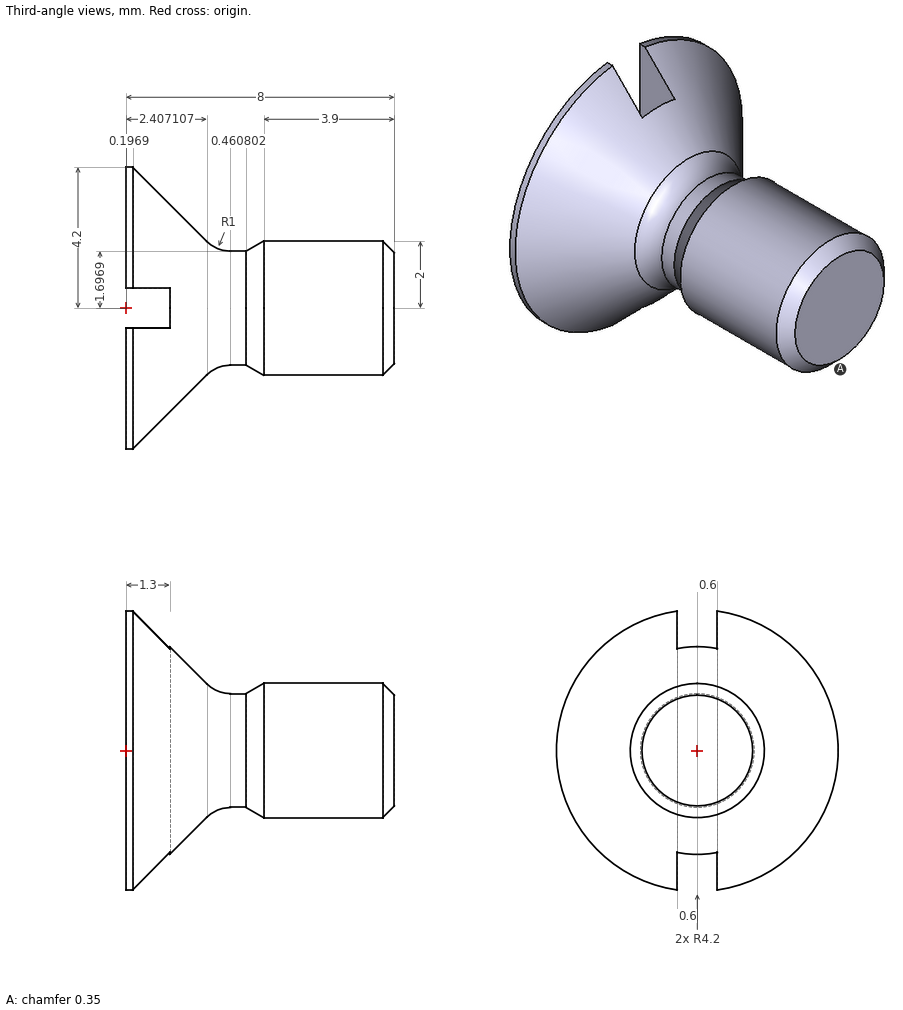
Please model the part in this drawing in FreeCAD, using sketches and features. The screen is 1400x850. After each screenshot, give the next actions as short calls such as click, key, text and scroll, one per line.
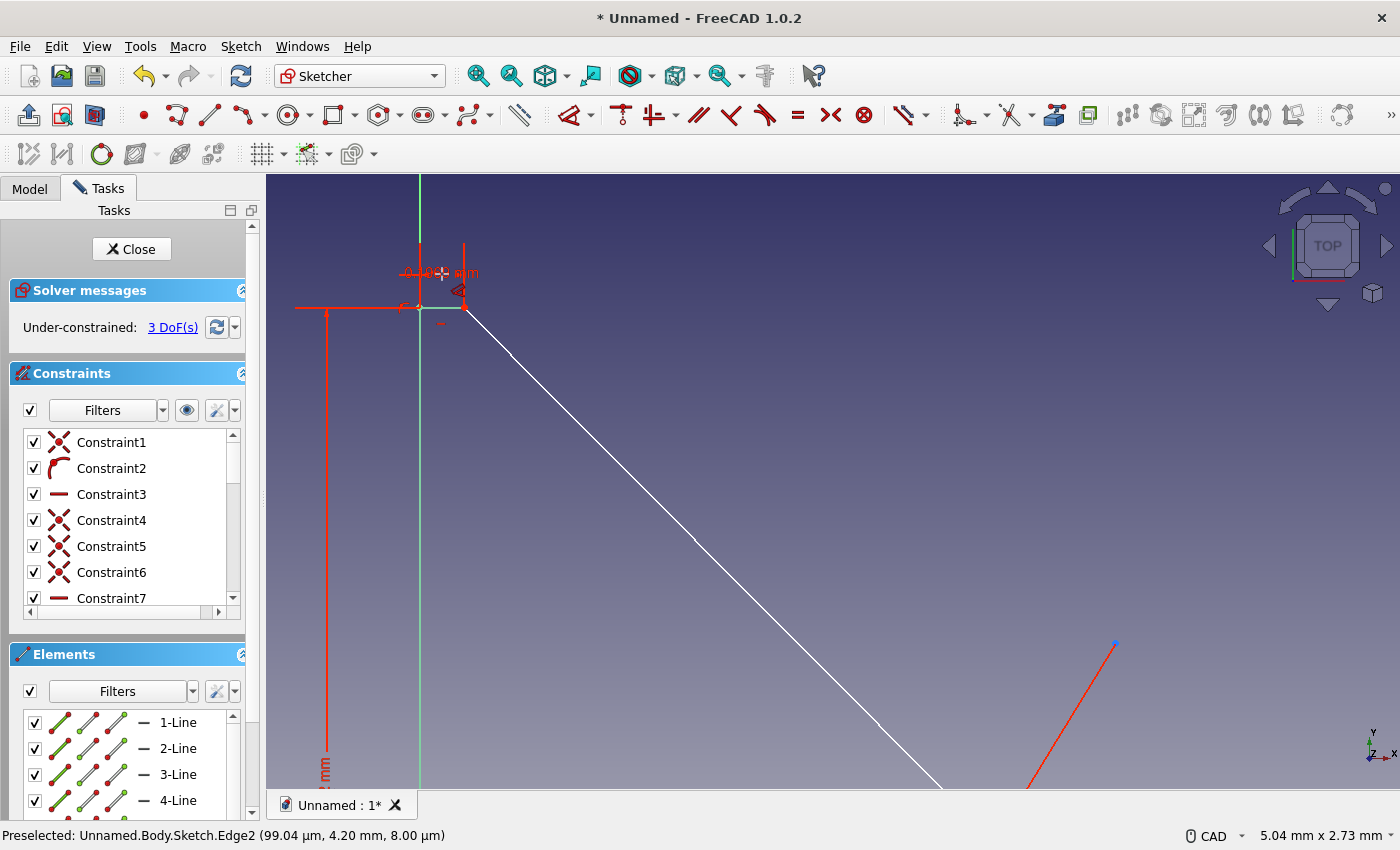
scroll(441, 308, down, 5)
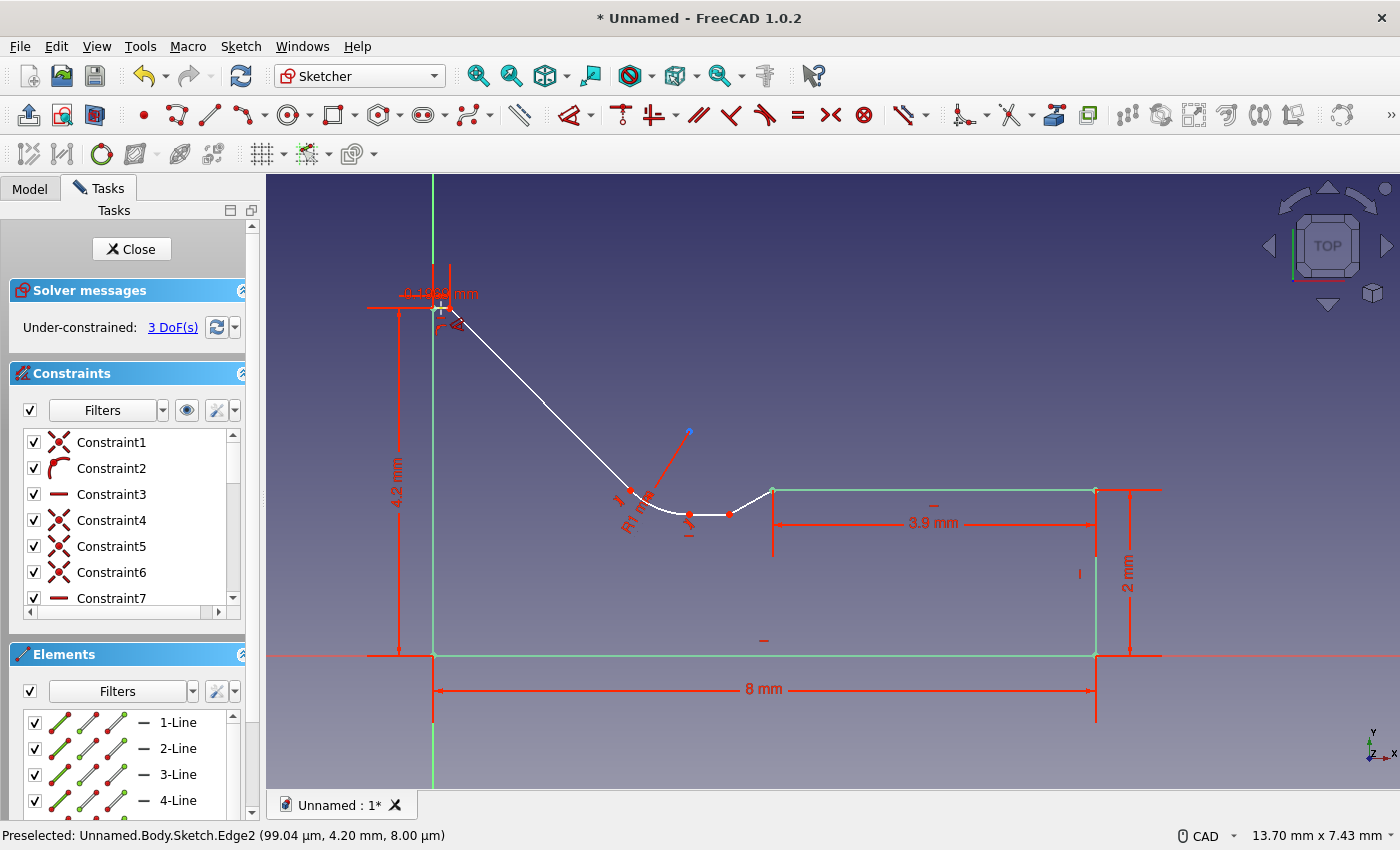
click(730, 515)
click(399, 585)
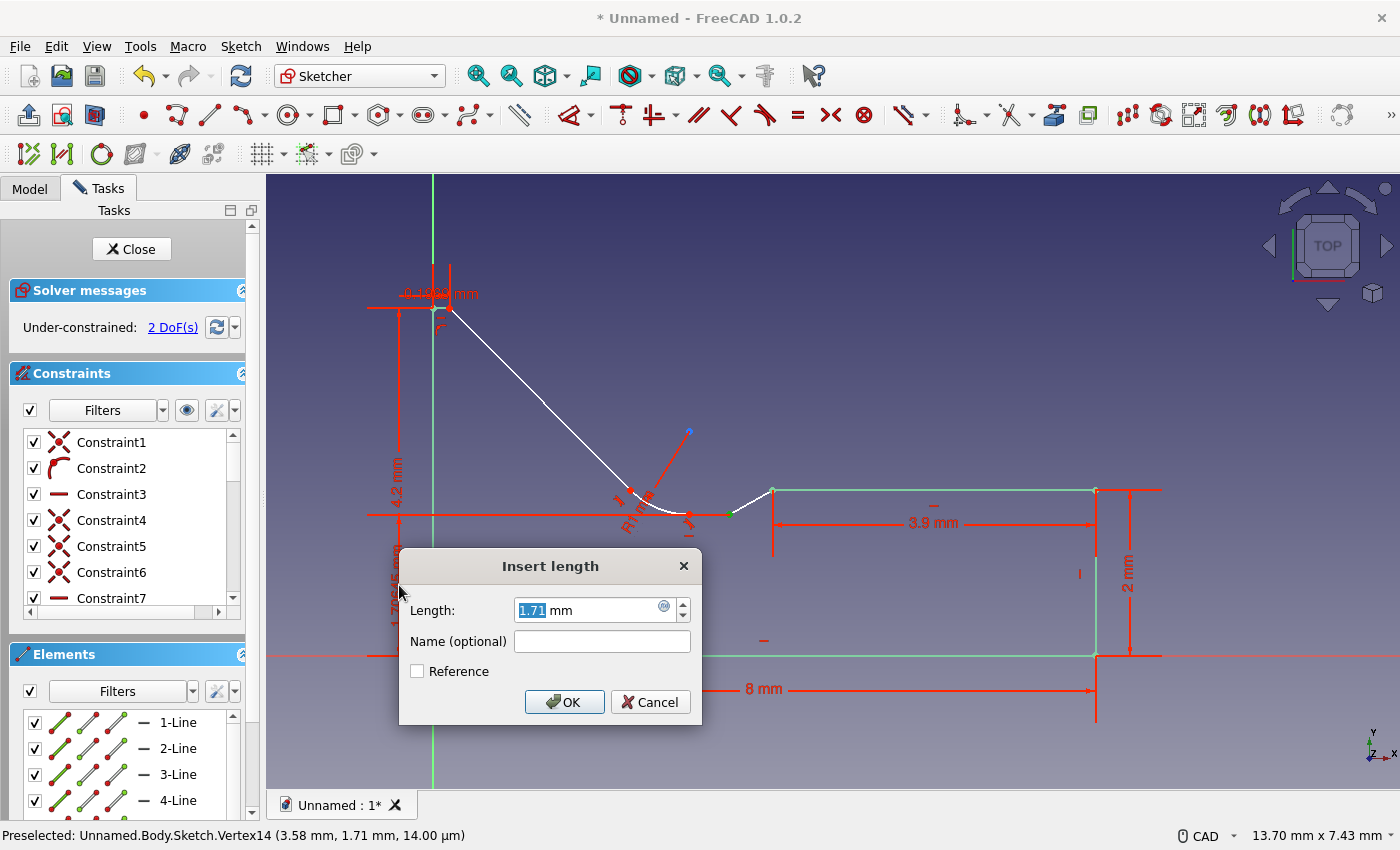
text(1.6969)
key(Return)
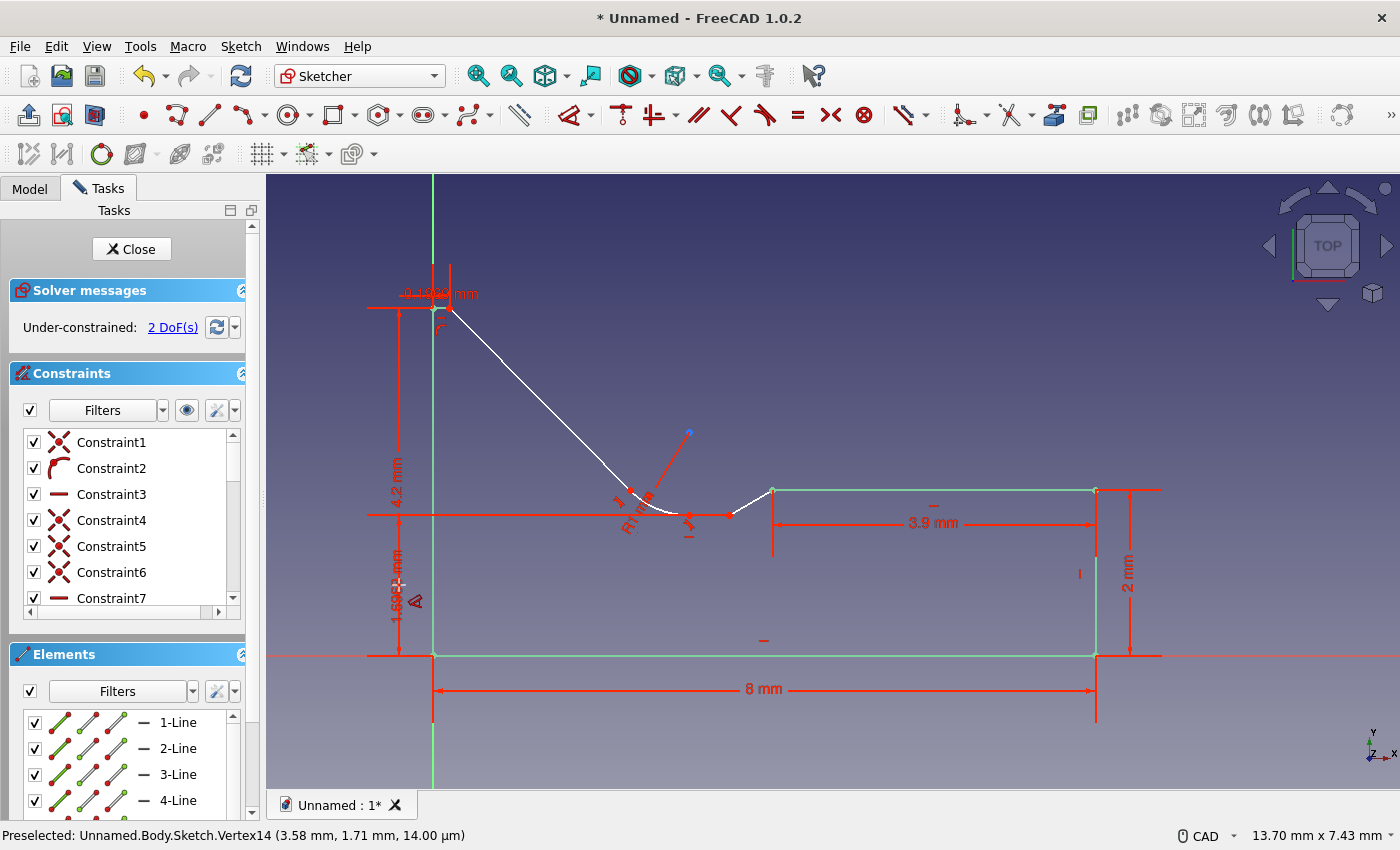
click(718, 515)
click(710, 549)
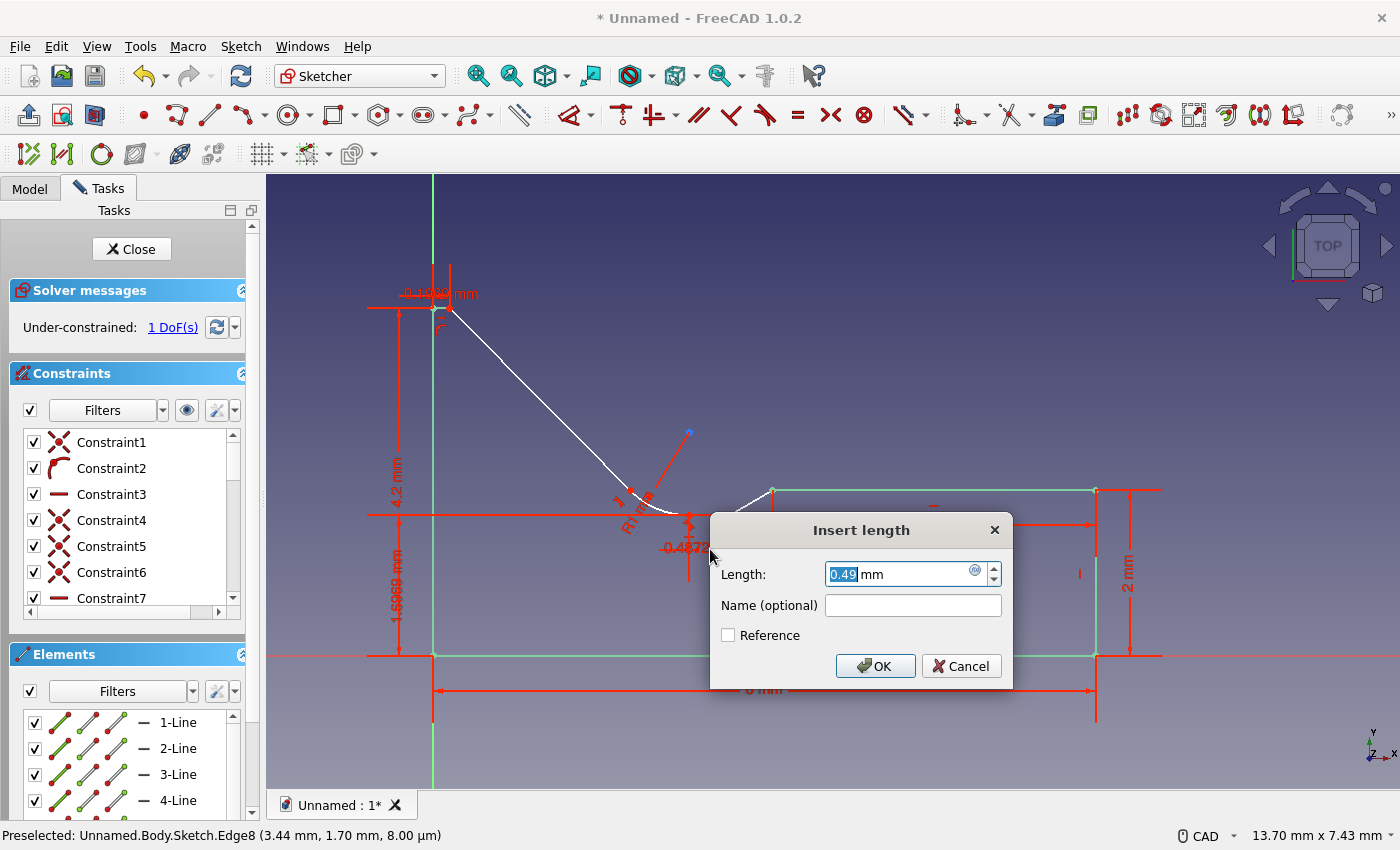
text(0.460802)
key(Return)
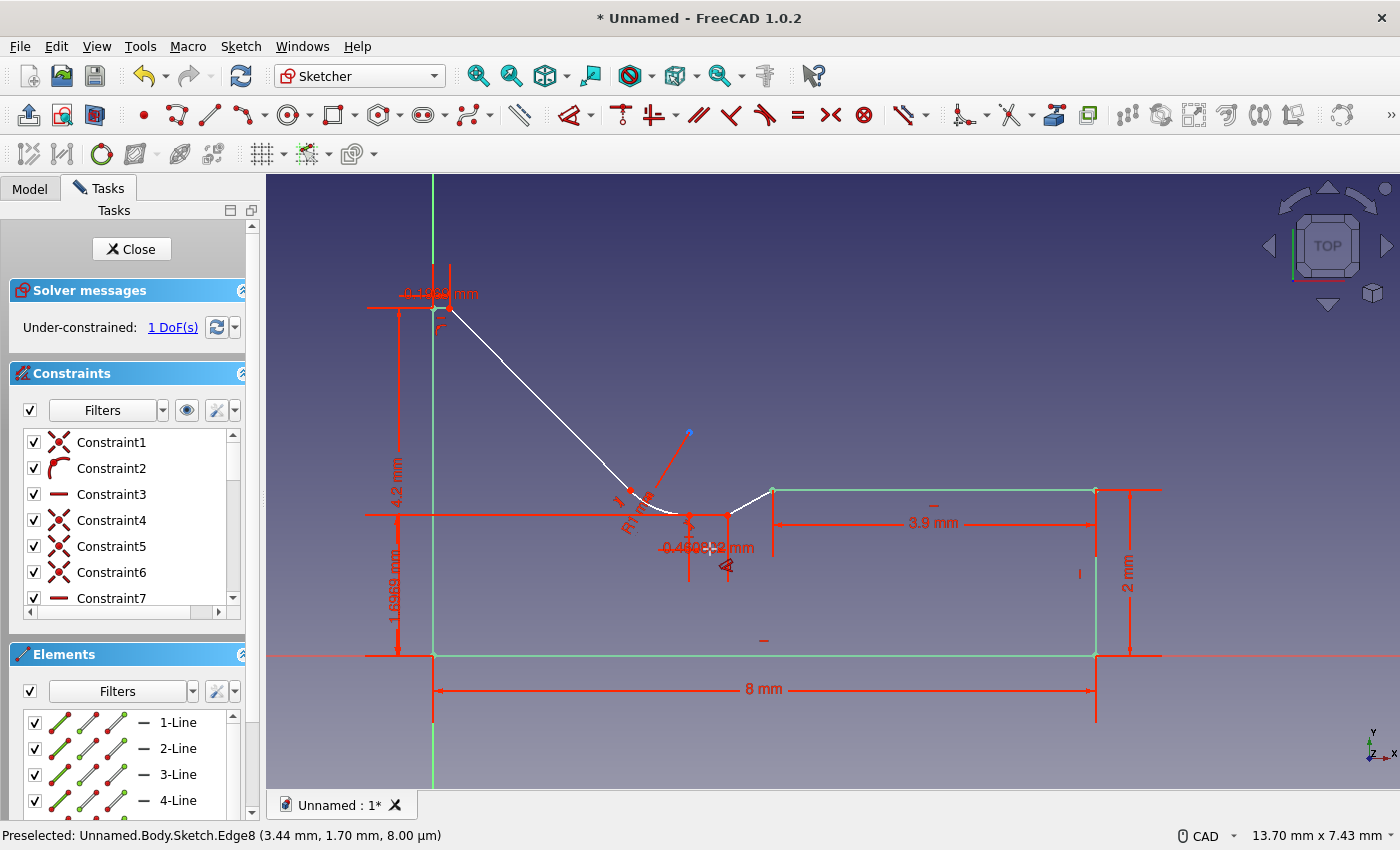
click(631, 491)
click(532, 690)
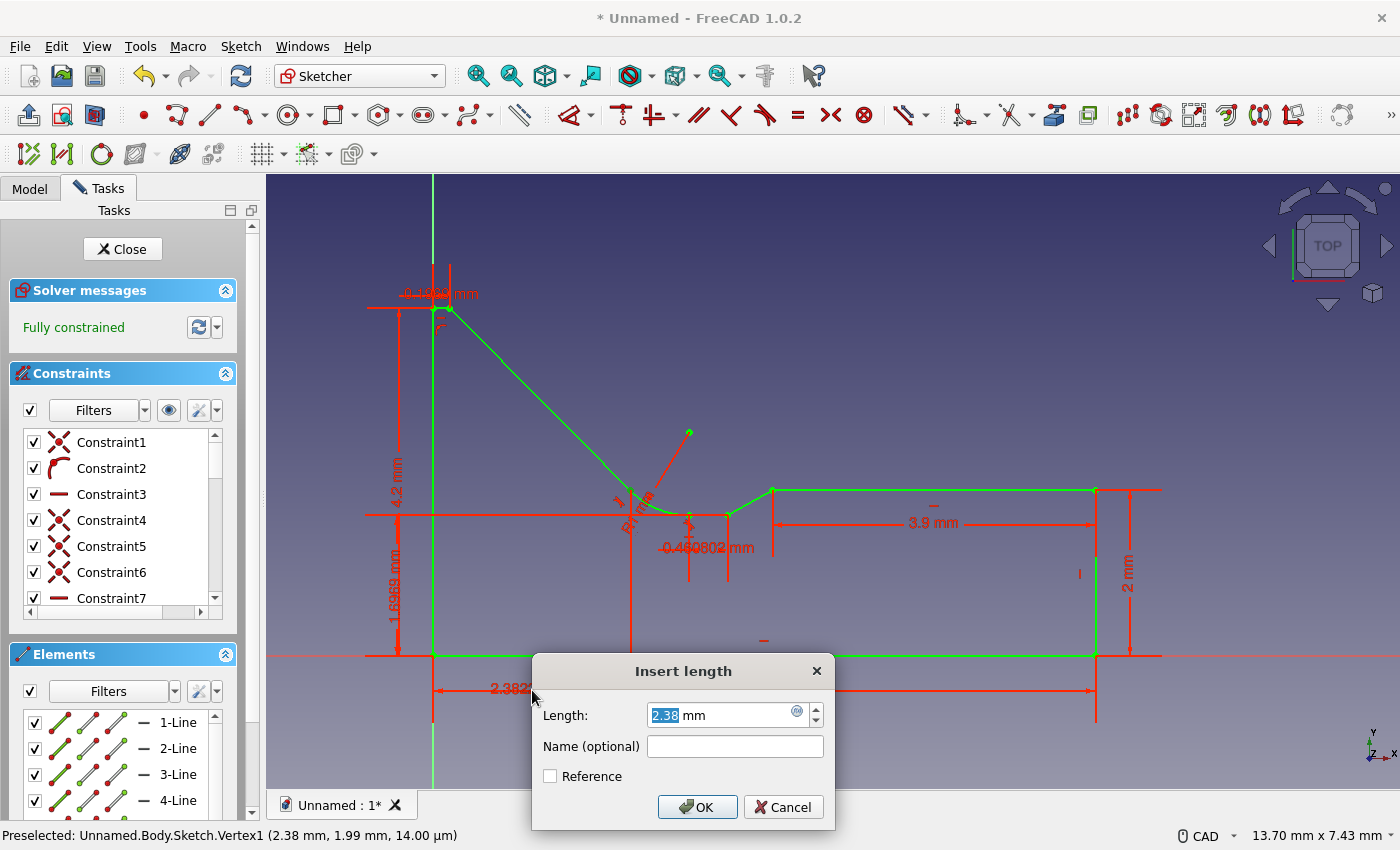
text(2.407107)
key(Return)
key(Escape)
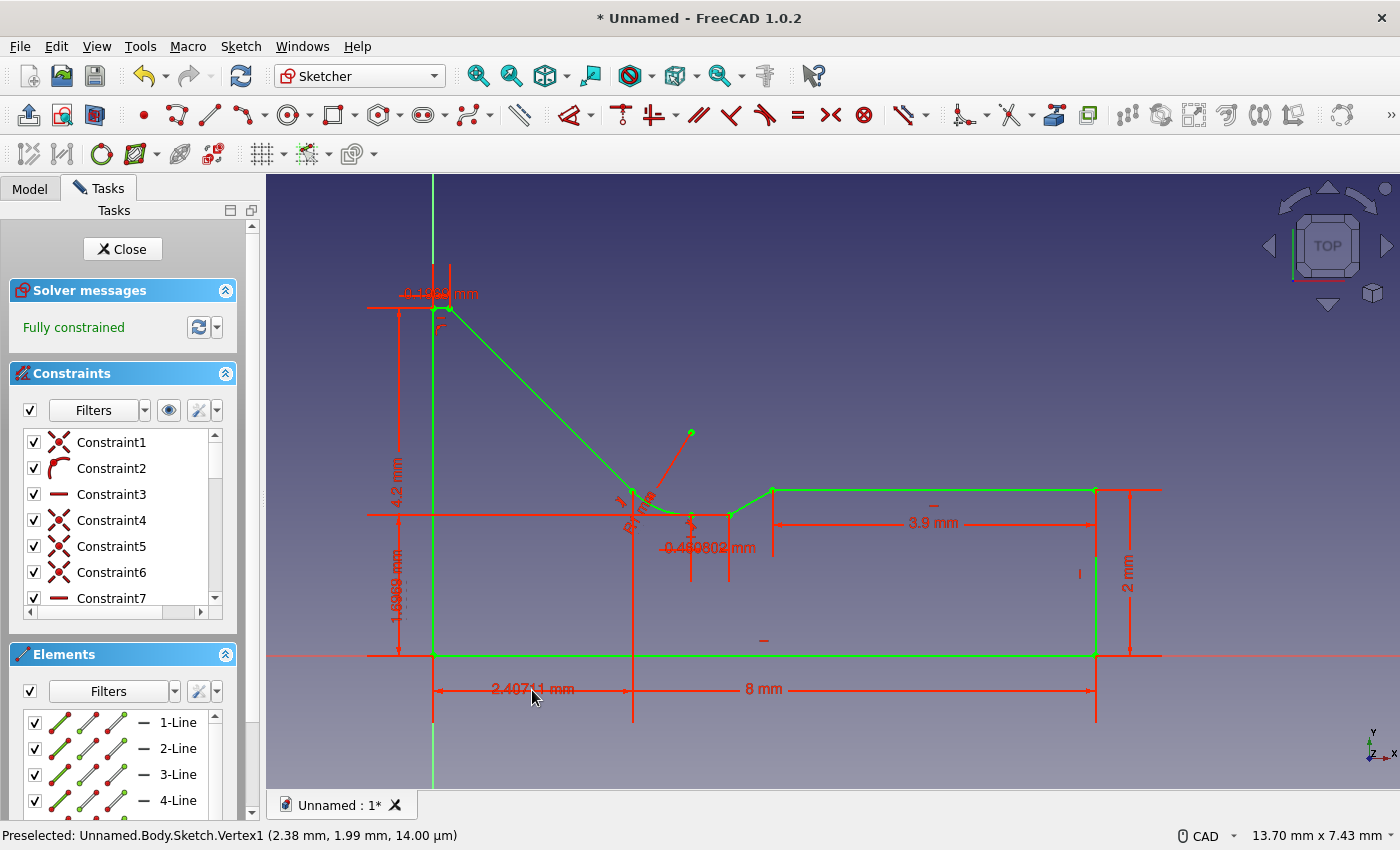
click(123, 249)